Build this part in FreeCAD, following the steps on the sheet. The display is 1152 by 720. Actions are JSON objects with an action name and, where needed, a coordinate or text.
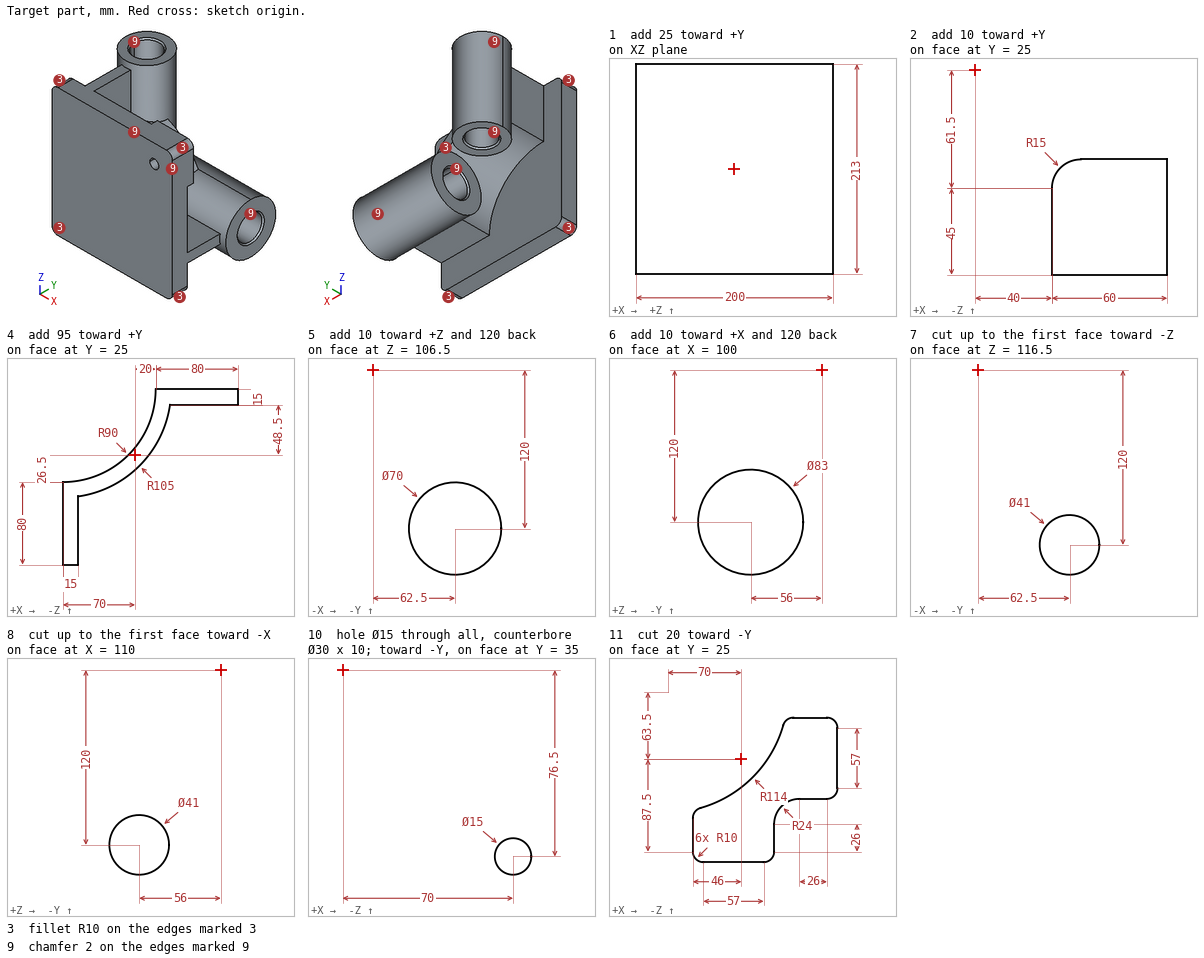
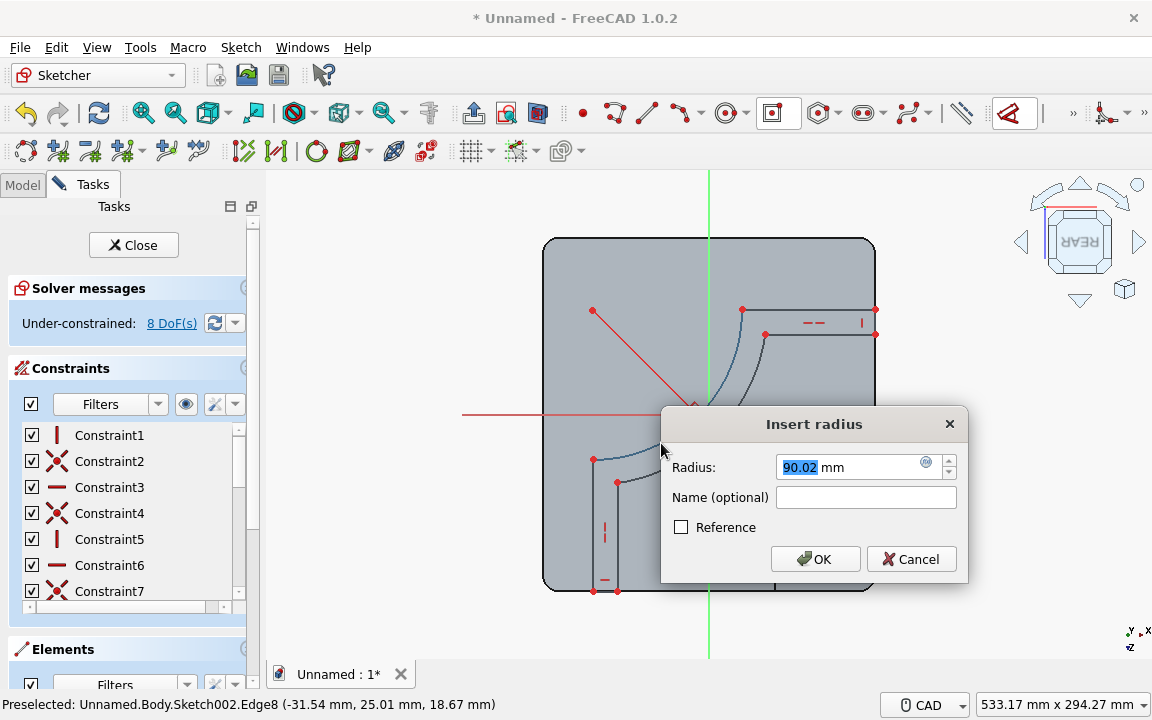
{"action": "type", "text": "90"}
{"action": "key", "text": "Return"}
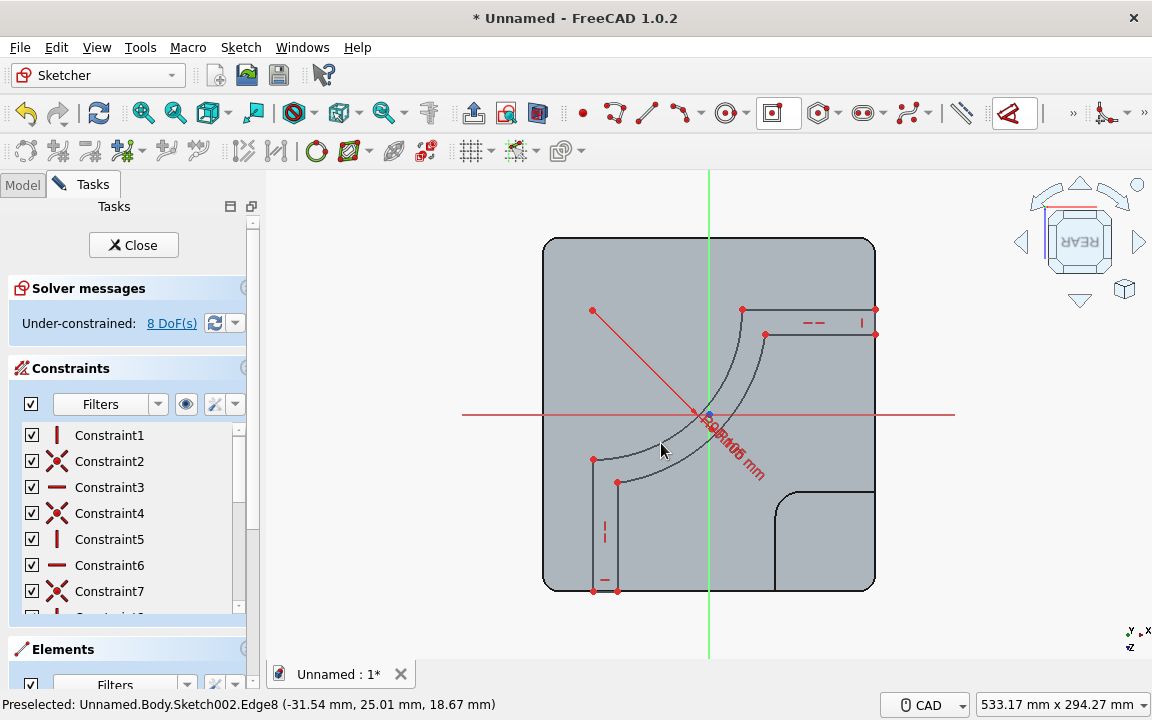
{"action": "left_click", "coordinate": [593, 500]}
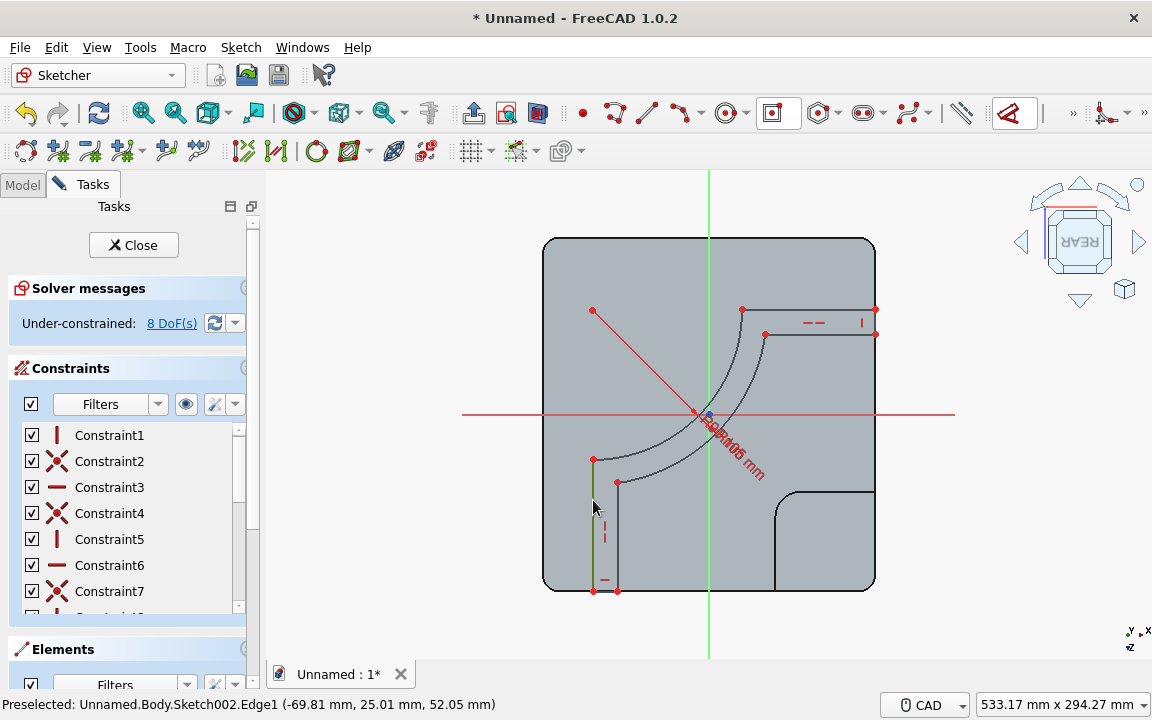
{"action": "left_click", "coordinate": [1032, 114]}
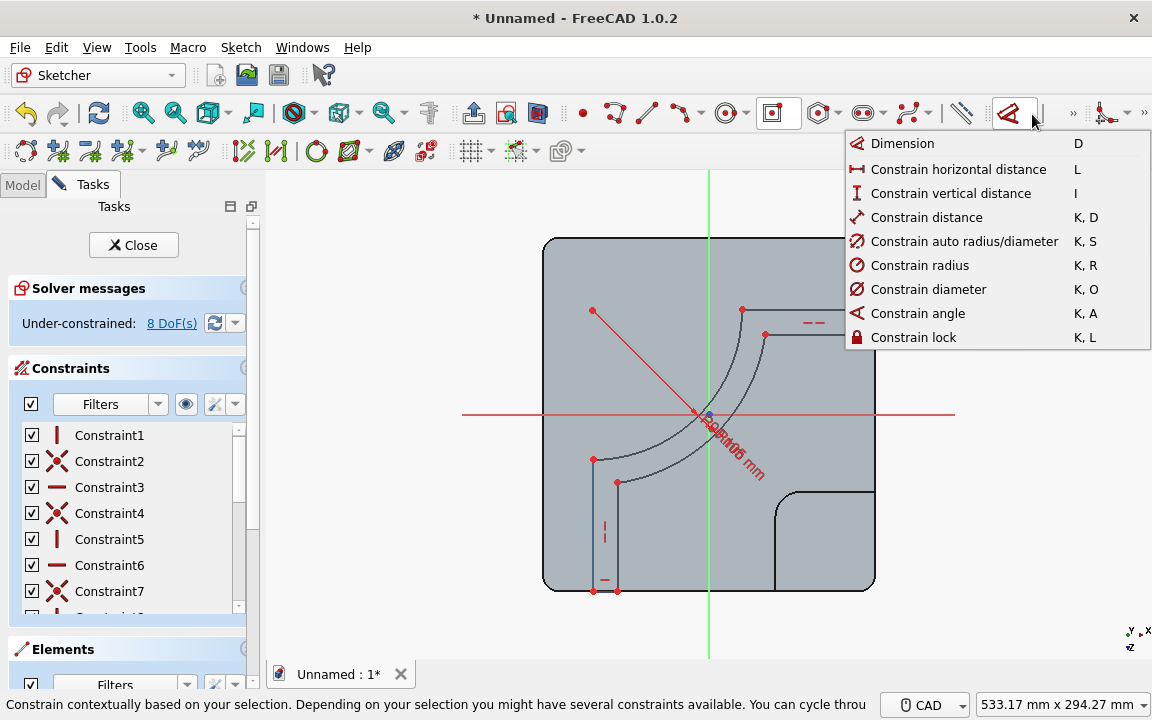
{"action": "left_click", "coordinate": [998, 193]}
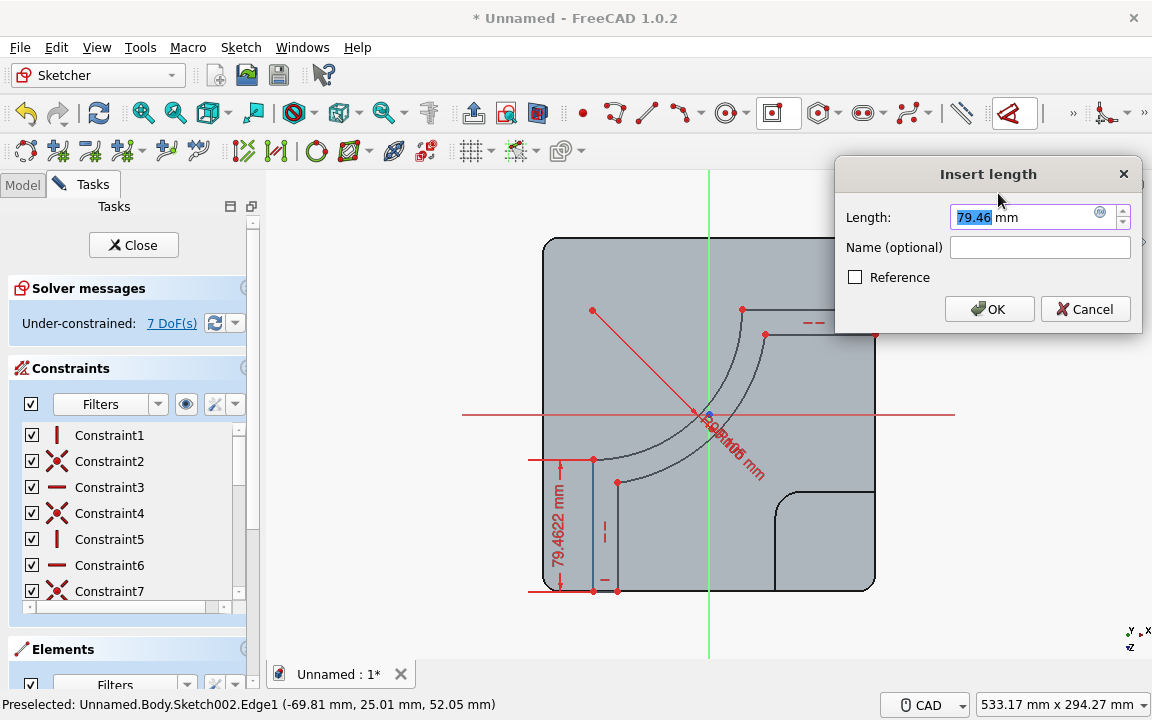
{"action": "type", "text": "80"}
{"action": "key", "text": "Return"}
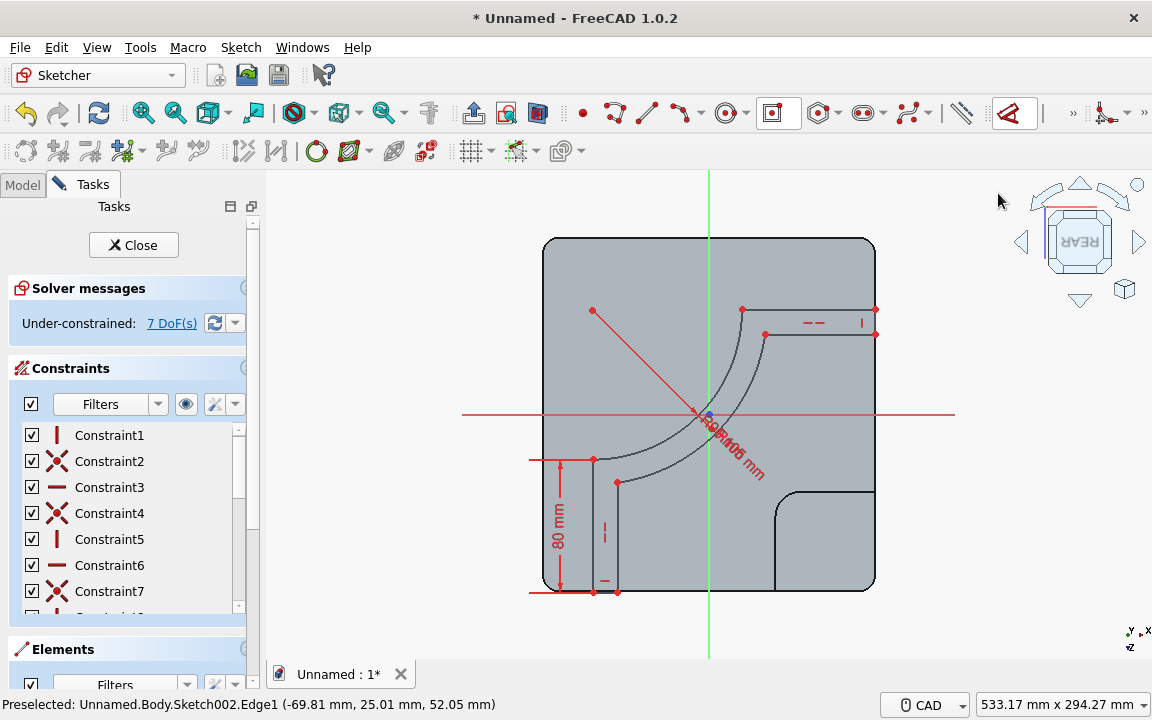
{"action": "scroll", "coordinate": [603, 593], "scroll_direction": "up", "scroll_amount": 3}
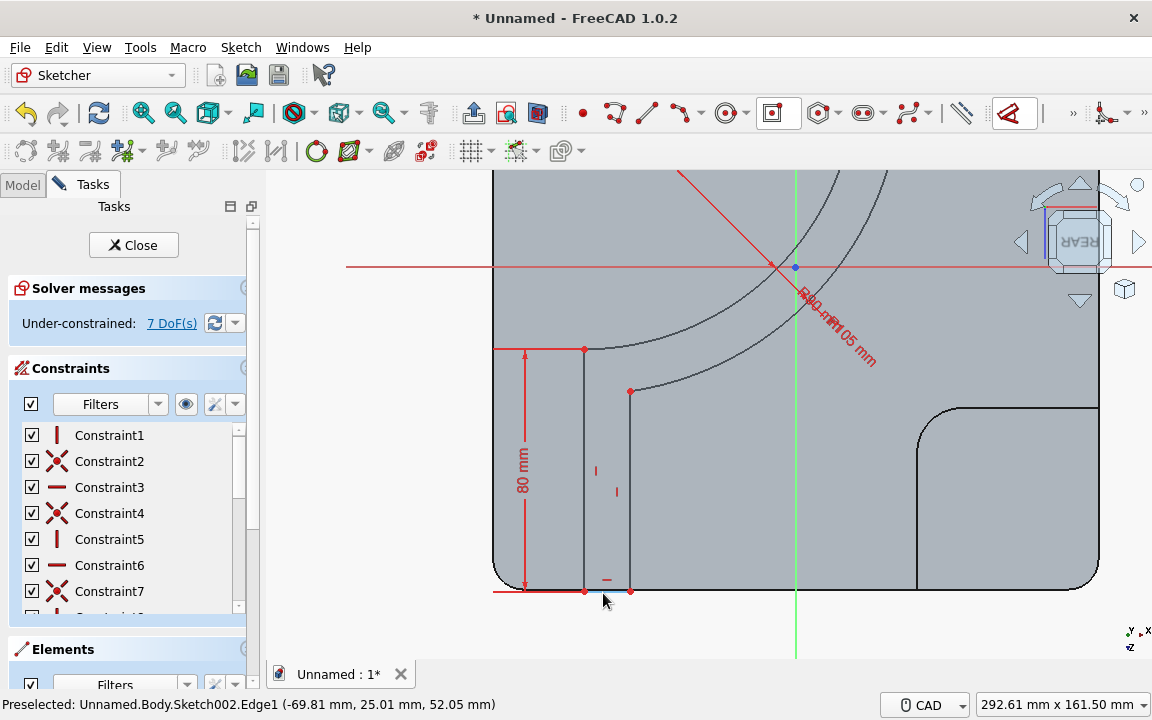
{"action": "left_click", "coordinate": [603, 592]}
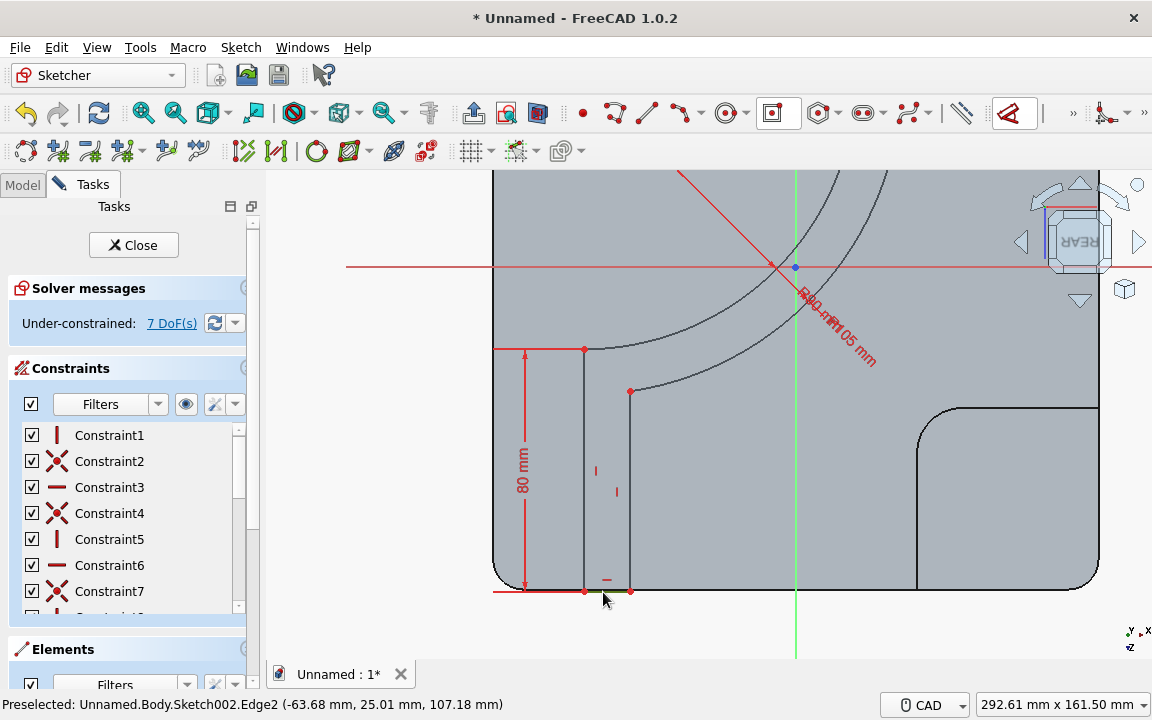
{"action": "left_click", "coordinate": [1032, 114]}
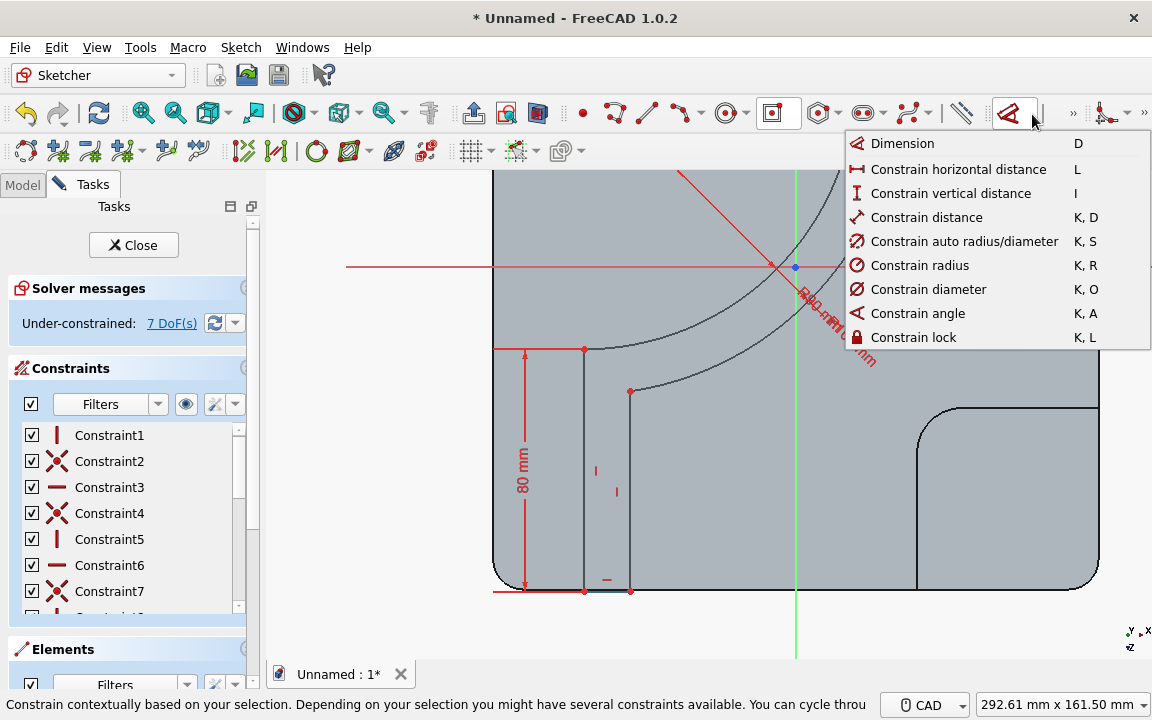
{"action": "left_click", "coordinate": [998, 169]}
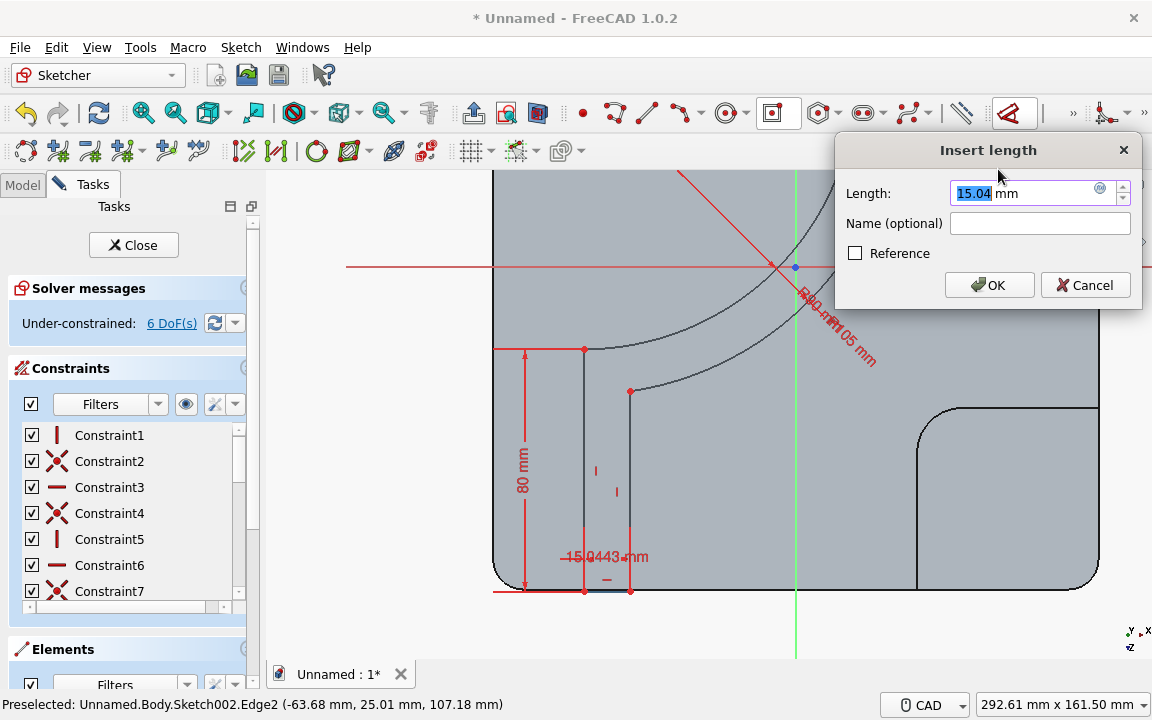
{"action": "type", "text": "15"}
{"action": "key", "text": "Return"}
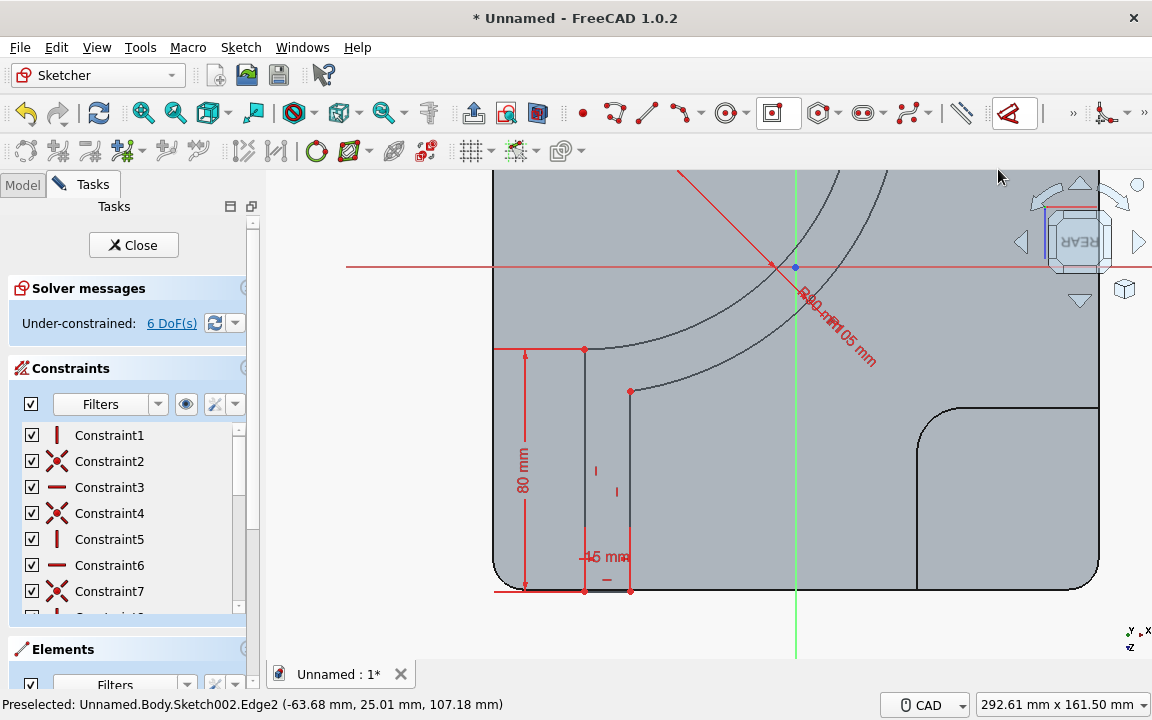
{"action": "scroll", "coordinate": [396, 515], "scroll_direction": "down", "scroll_amount": 3}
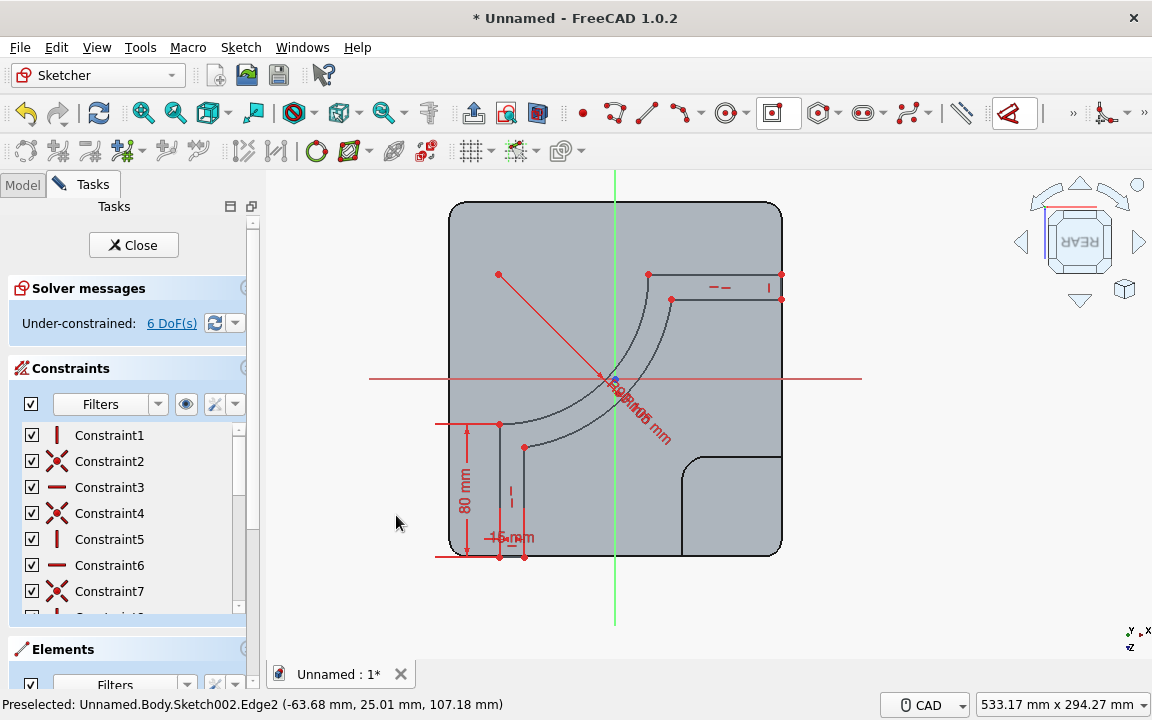
{"action": "scroll", "coordinate": [781, 292], "scroll_direction": "up", "scroll_amount": 4}